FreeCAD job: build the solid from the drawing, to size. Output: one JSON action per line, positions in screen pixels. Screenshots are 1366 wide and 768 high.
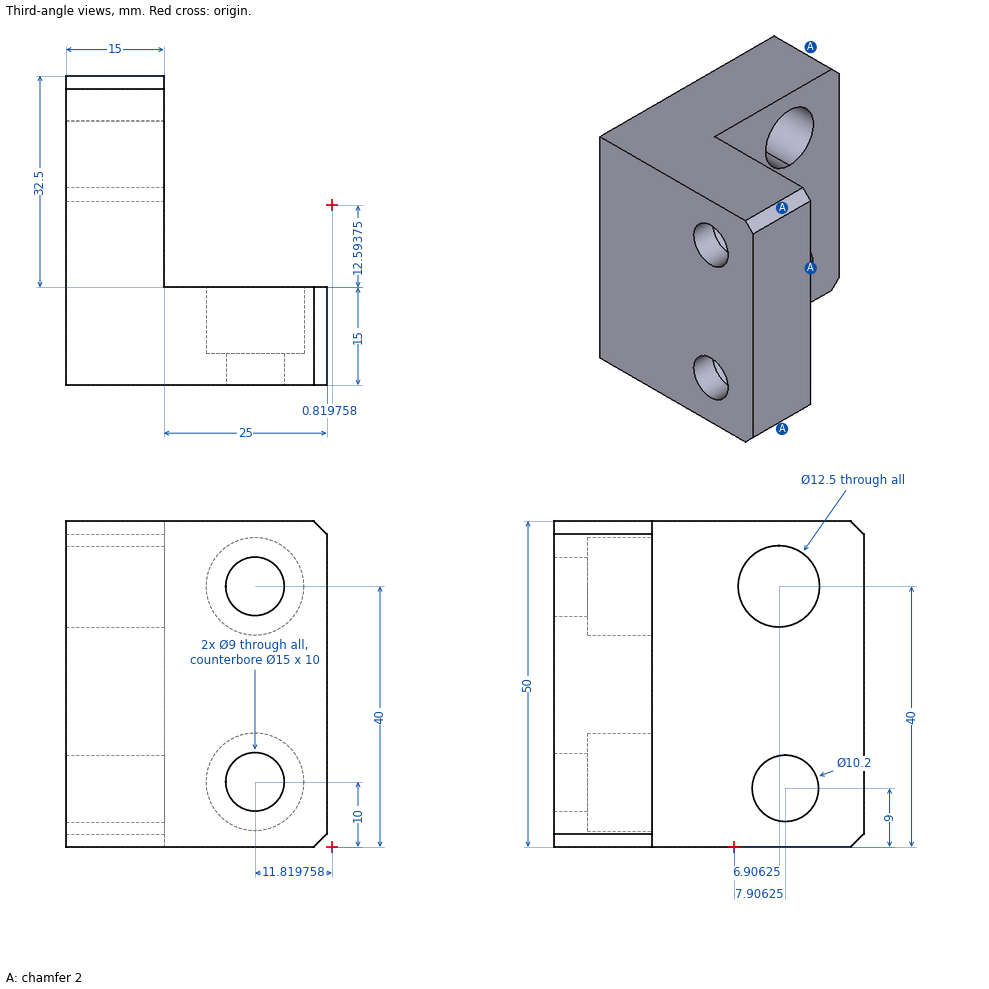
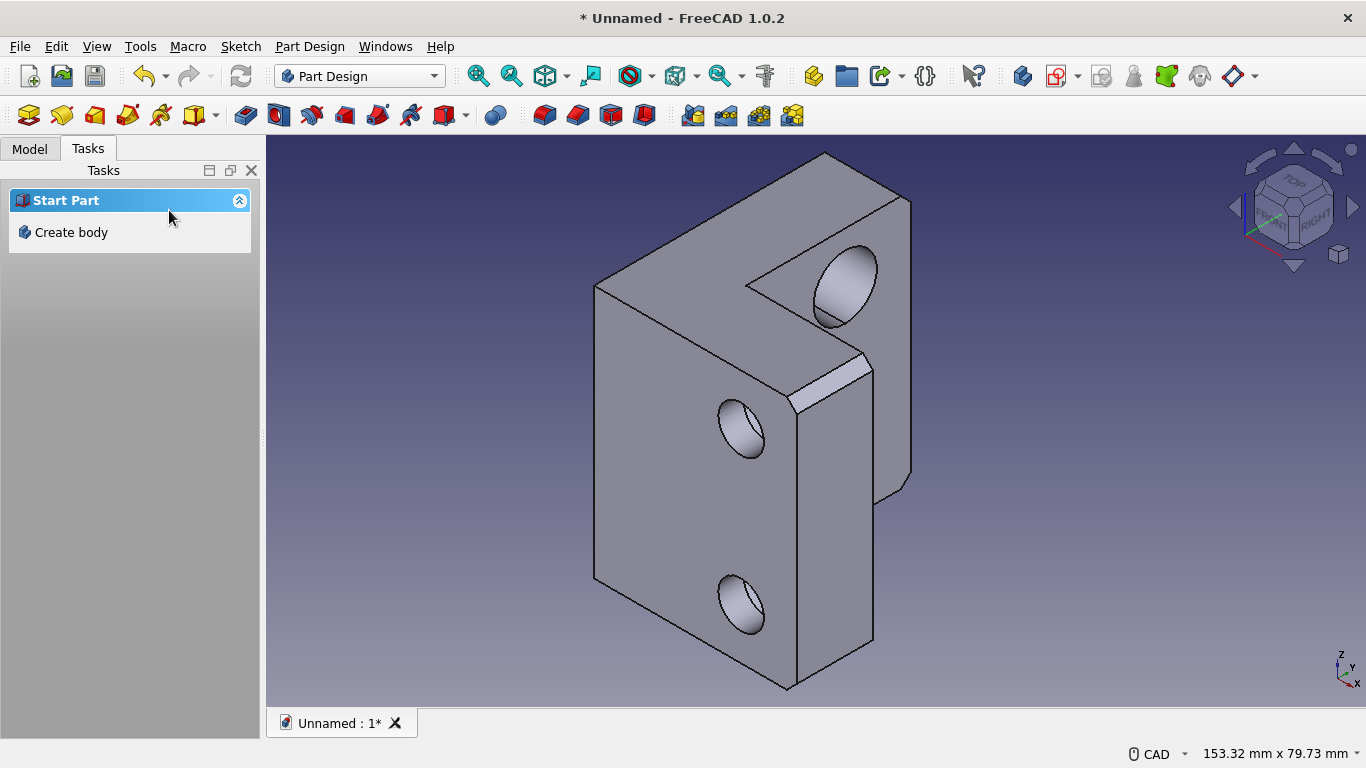
{"action": "key", "text": "3"}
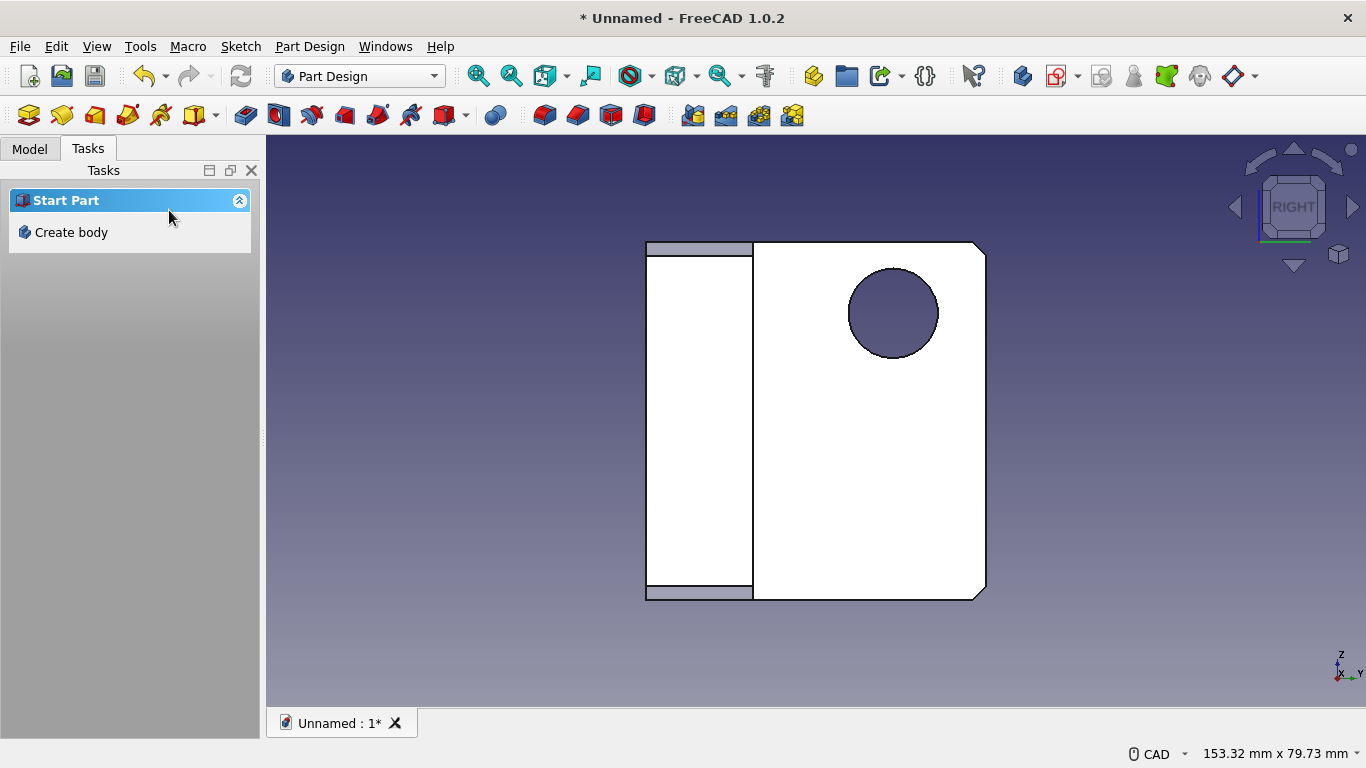
{"action": "left_click", "coordinate": [870, 471]}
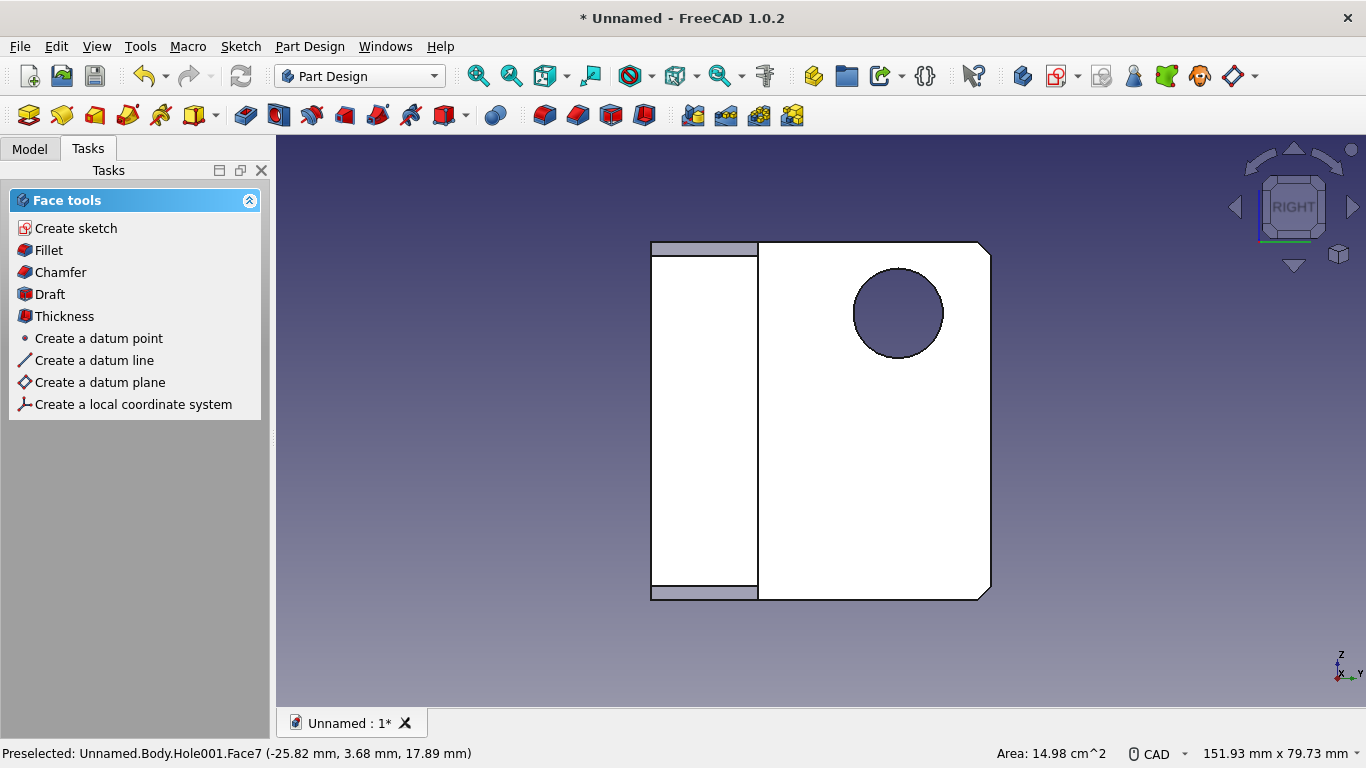
{"action": "left_click", "coordinate": [1056, 76]}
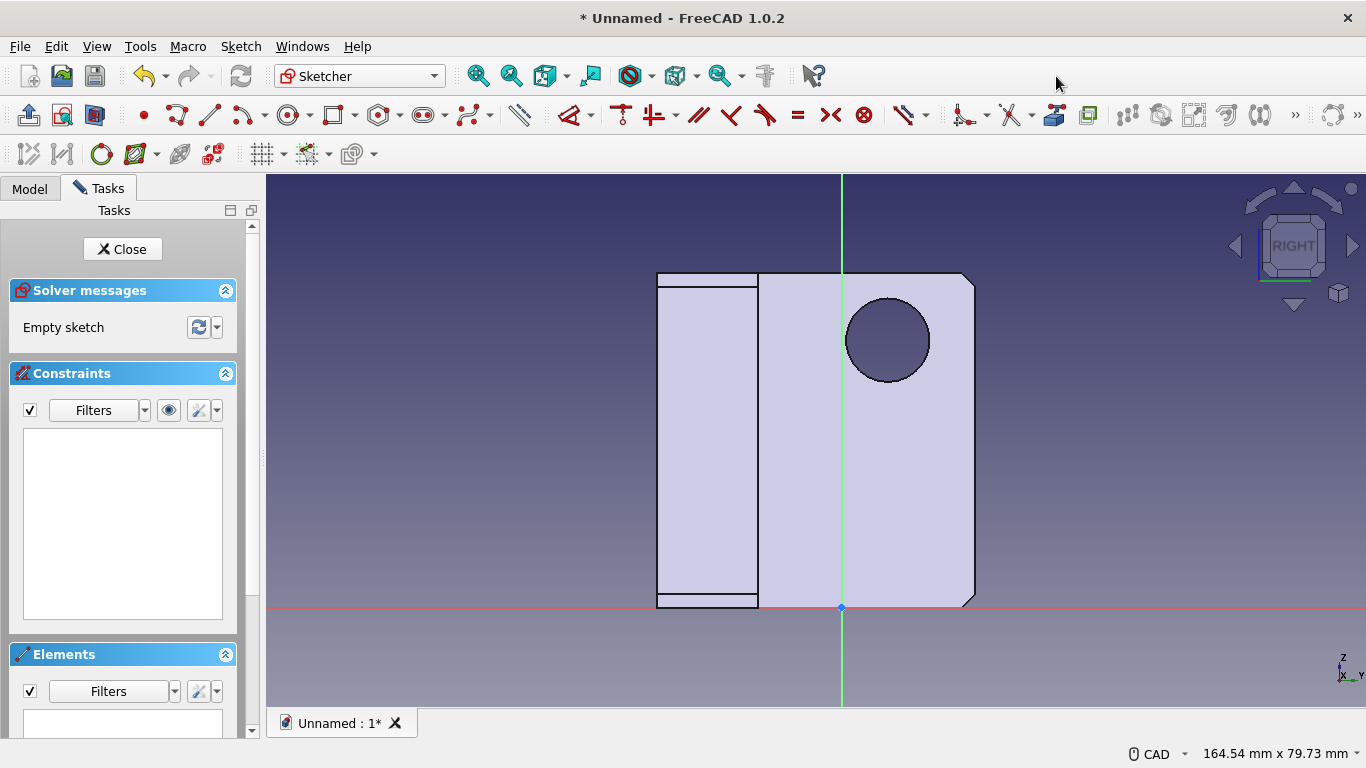
{"action": "left_click", "coordinate": [95, 116]}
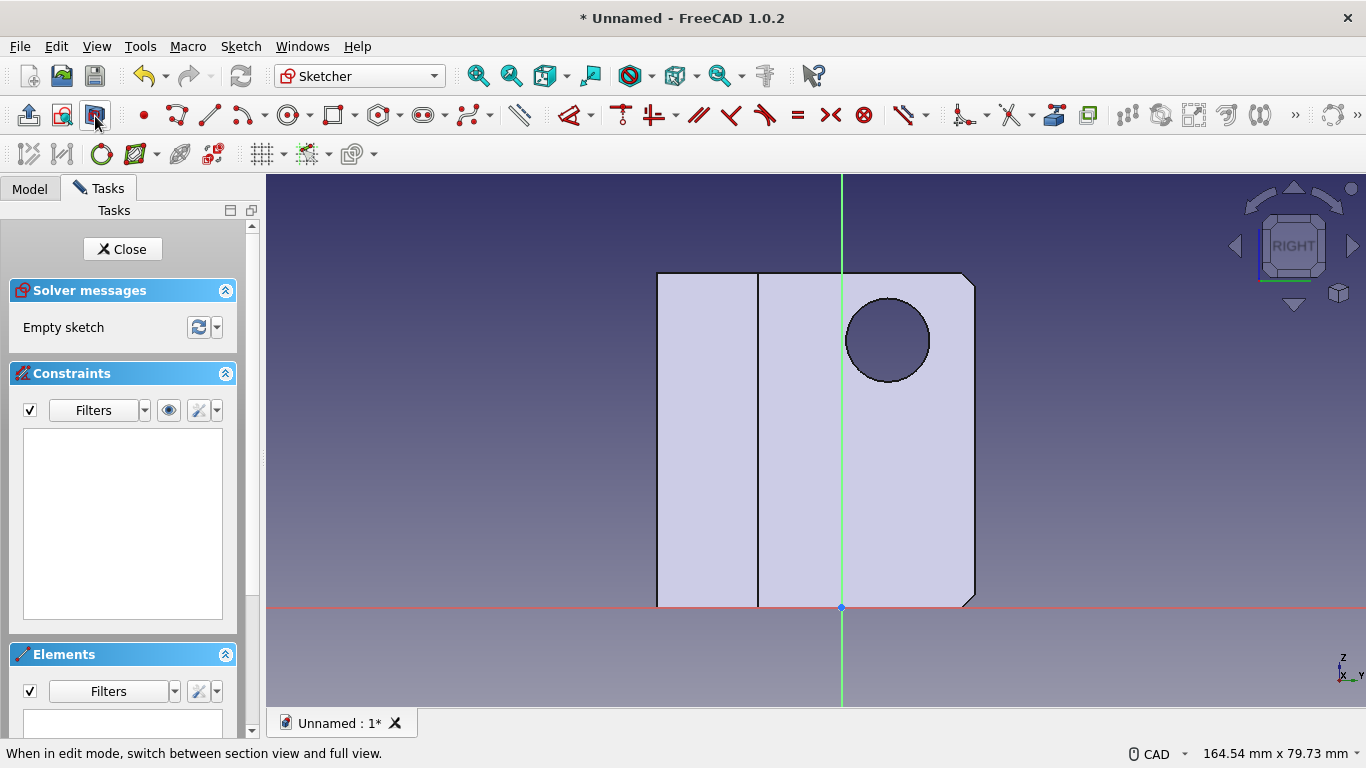
{"action": "scroll", "coordinate": [945, 612], "scroll_direction": "up", "scroll_amount": 6}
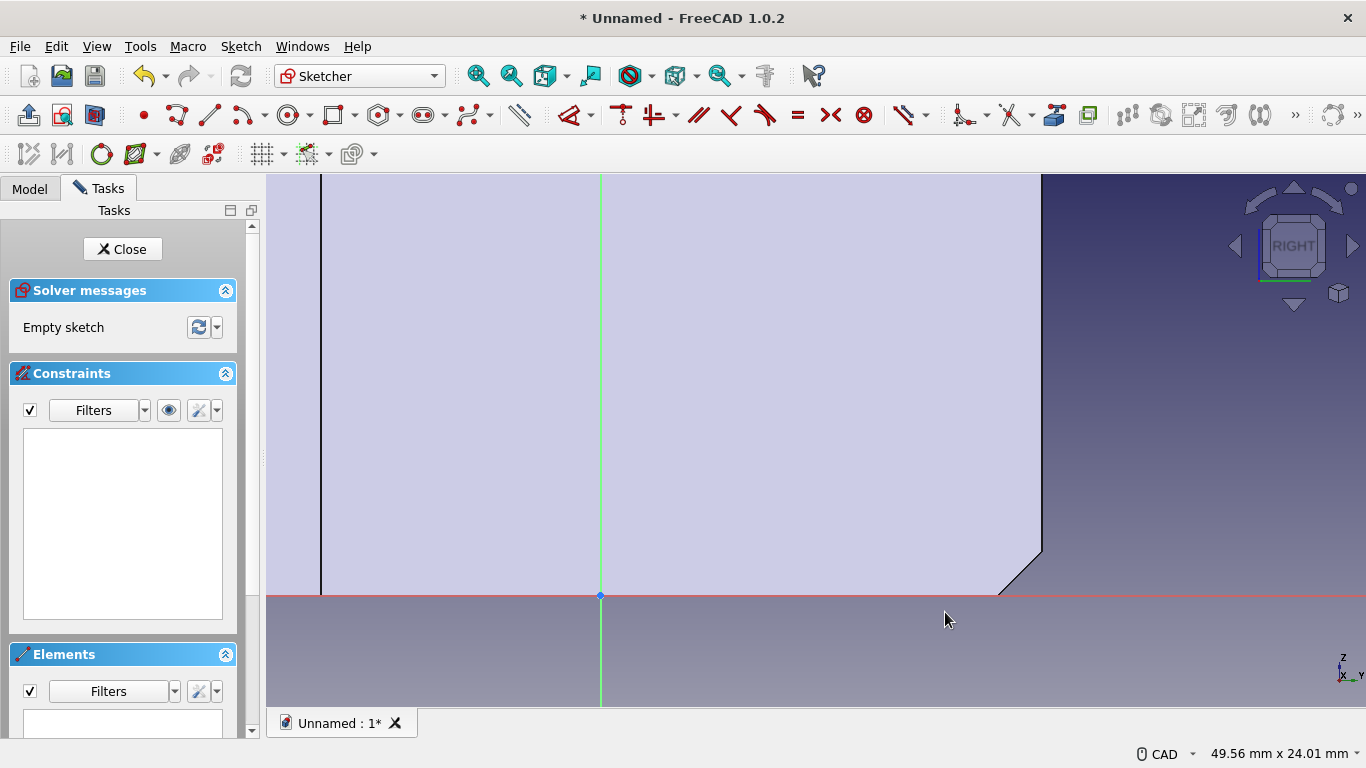
{"action": "left_click", "coordinate": [288, 116]}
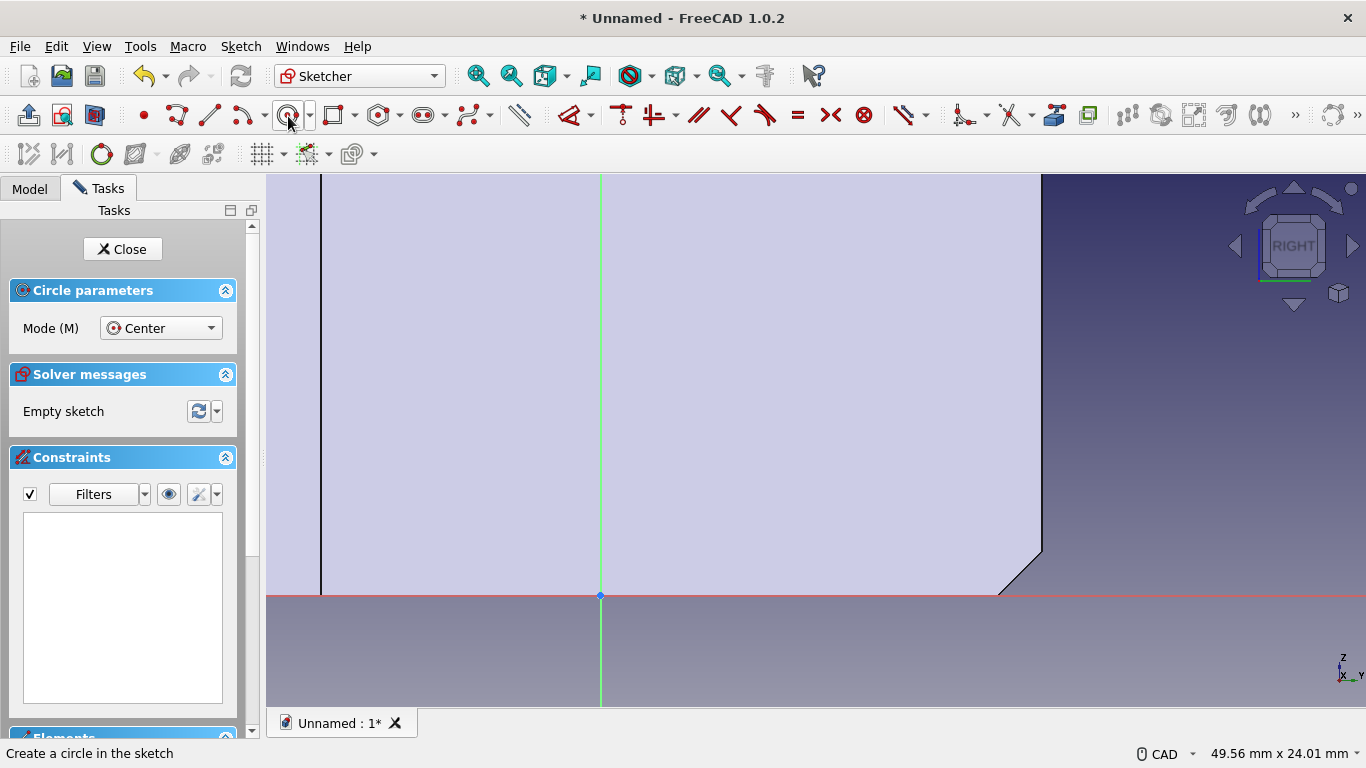
{"action": "left_click", "coordinate": [776, 396]}
{"action": "left_click", "coordinate": [856, 316]}
{"action": "key", "text": "Escape"}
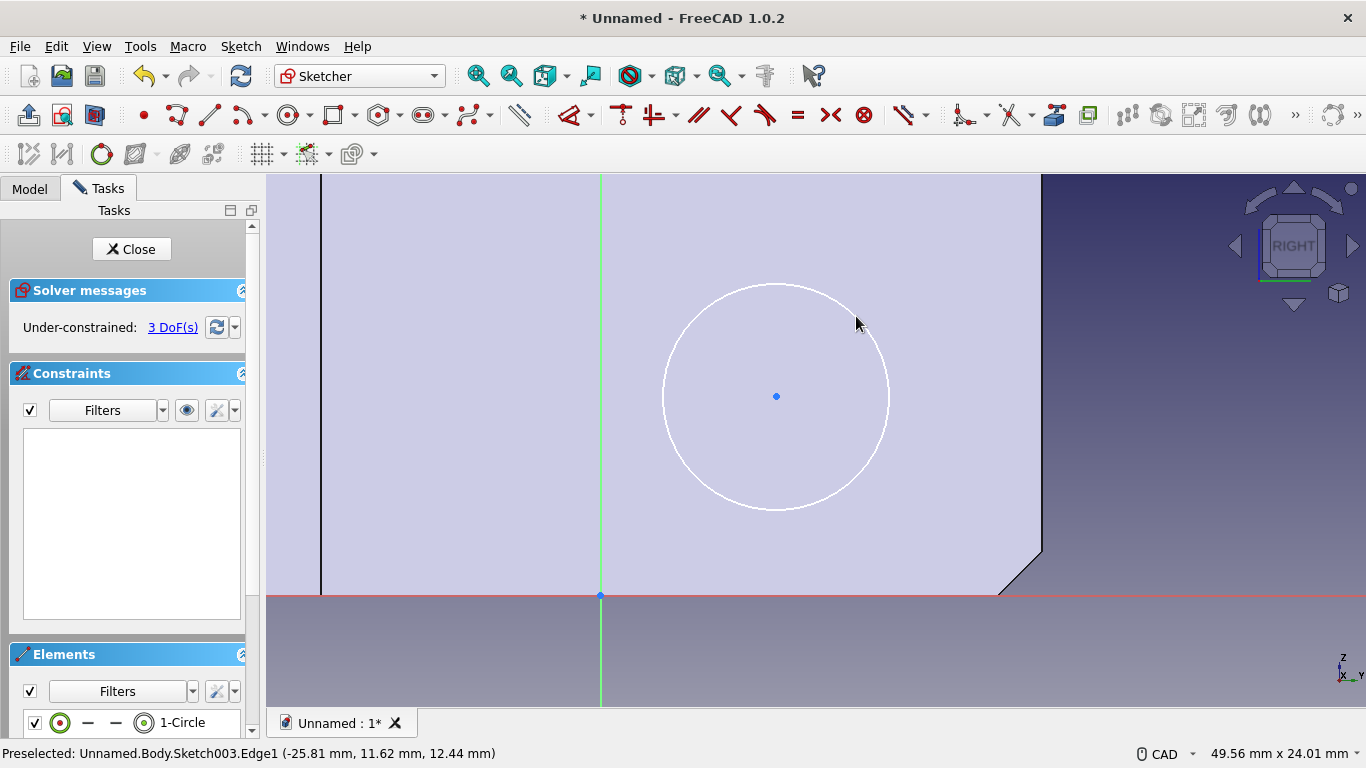
{"action": "left_click", "coordinate": [568, 116]}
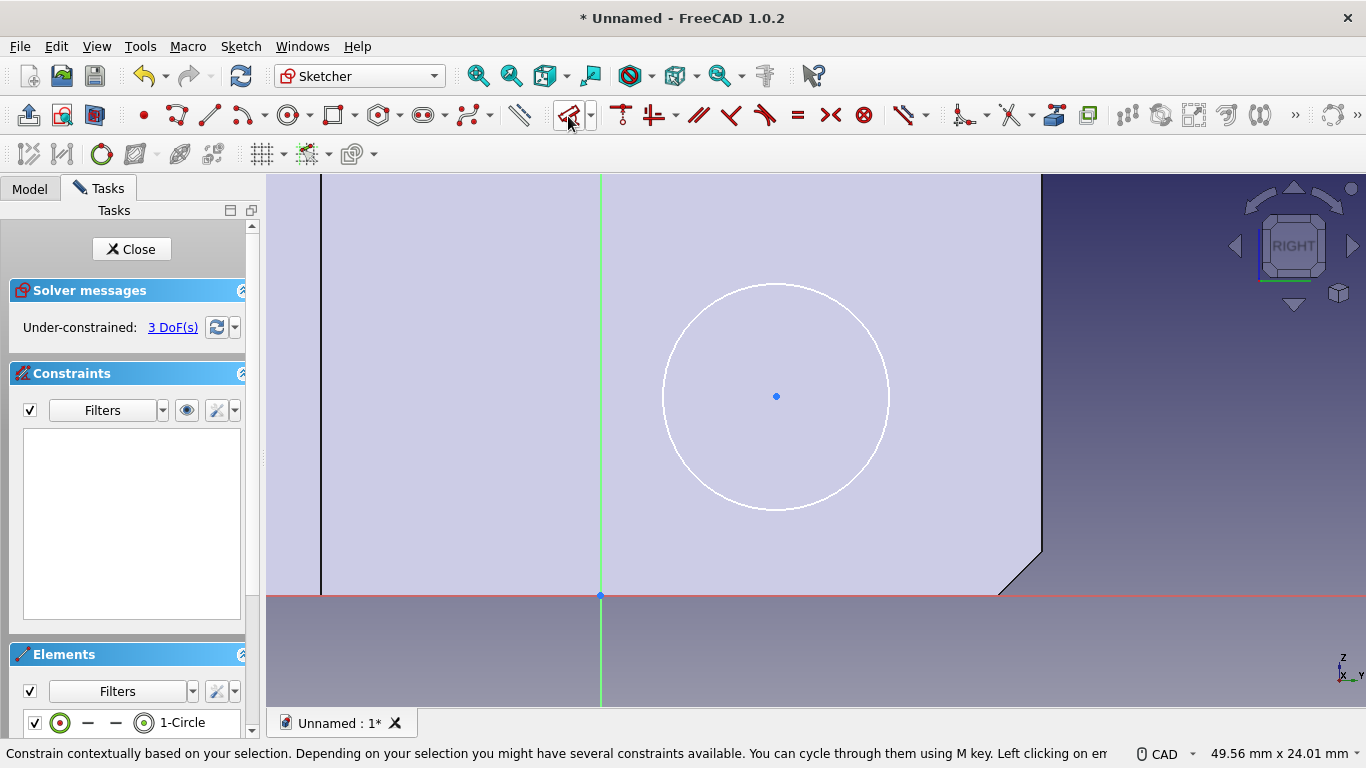
{"action": "left_click", "coordinate": [856, 317]}
{"action": "left_click", "coordinate": [879, 294]}